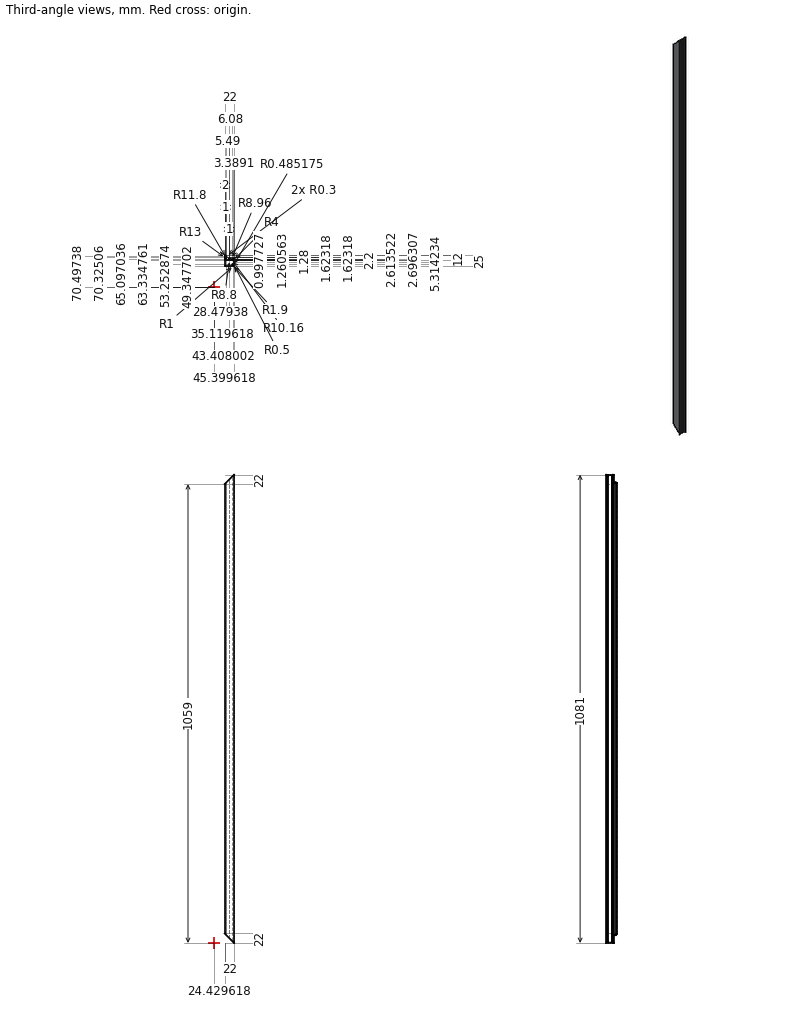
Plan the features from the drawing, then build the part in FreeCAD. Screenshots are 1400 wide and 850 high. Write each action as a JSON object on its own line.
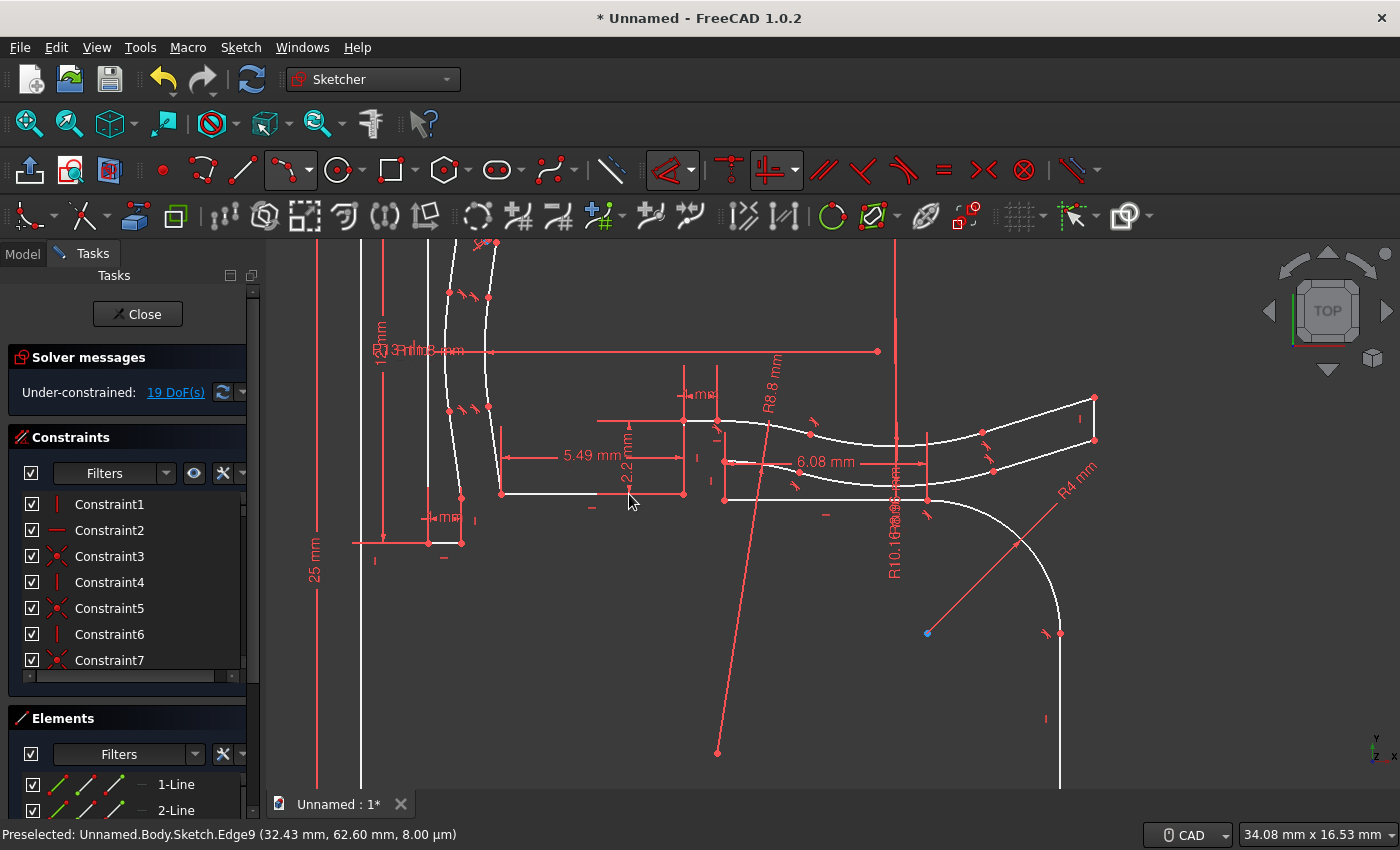
{"action": "left_click", "coordinate": [461, 530]}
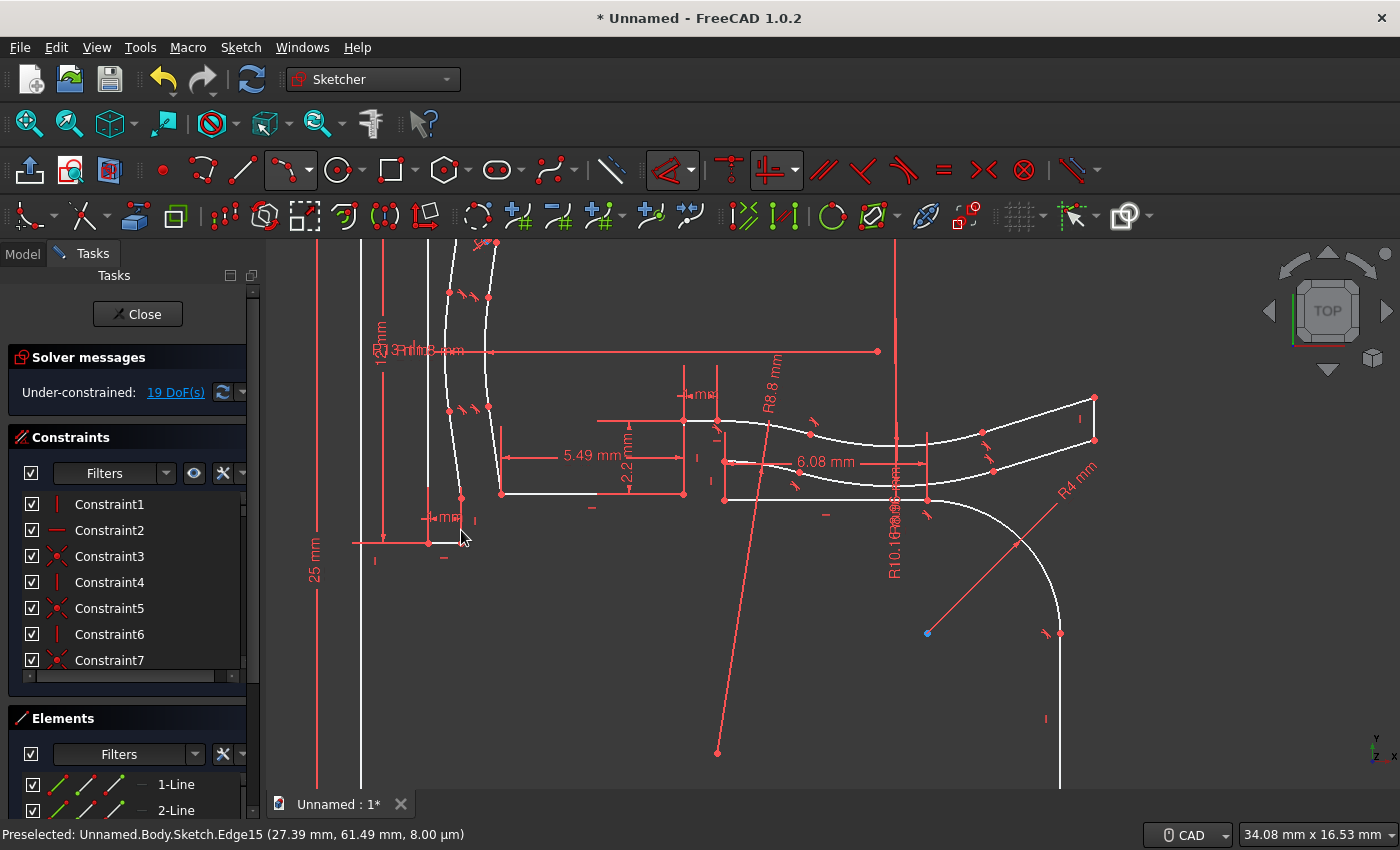
{"action": "left_click", "coordinate": [694, 170]}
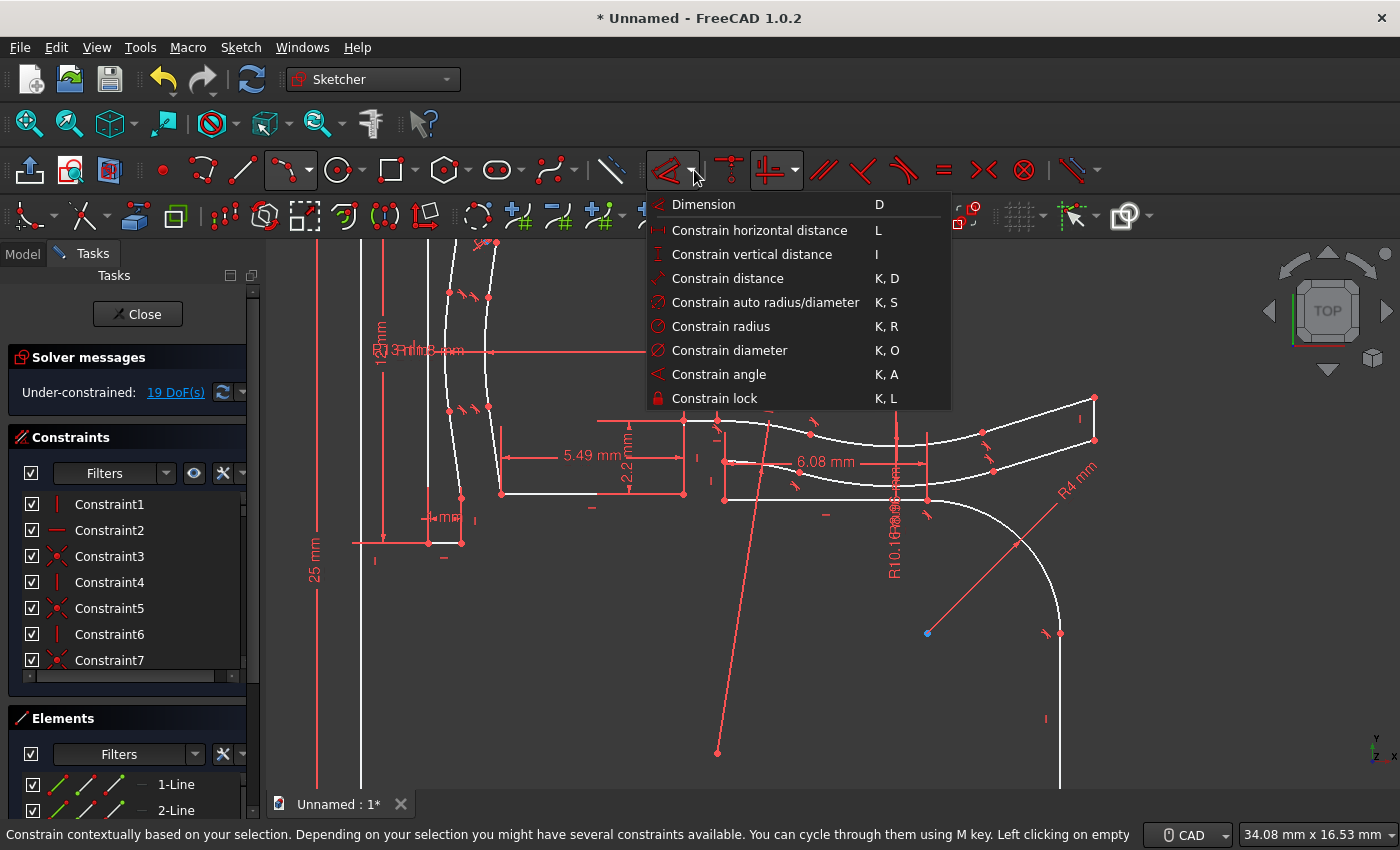
{"action": "left_click", "coordinate": [799, 254]}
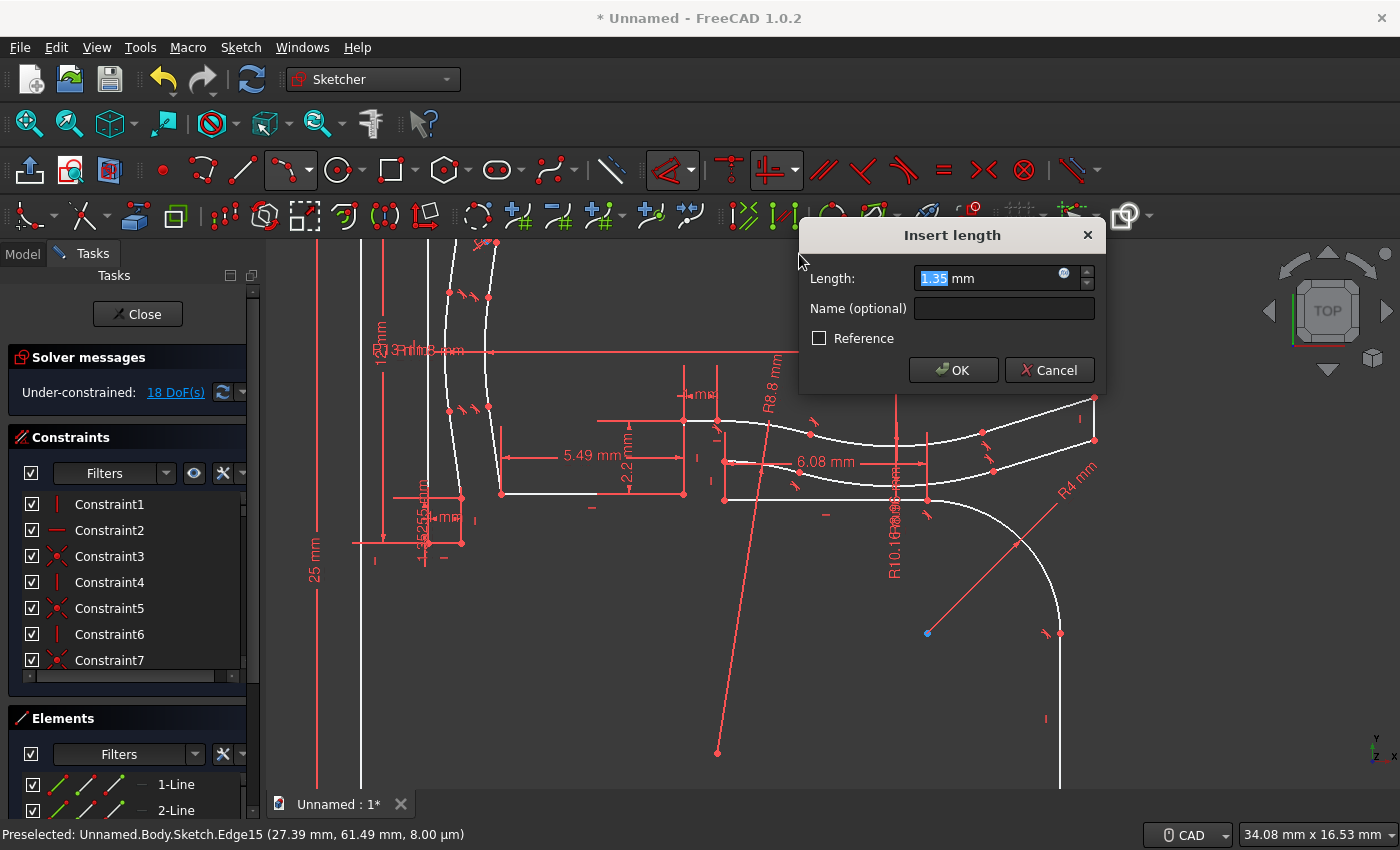
{"action": "type", "text": "1.28"}
{"action": "key", "text": "Return"}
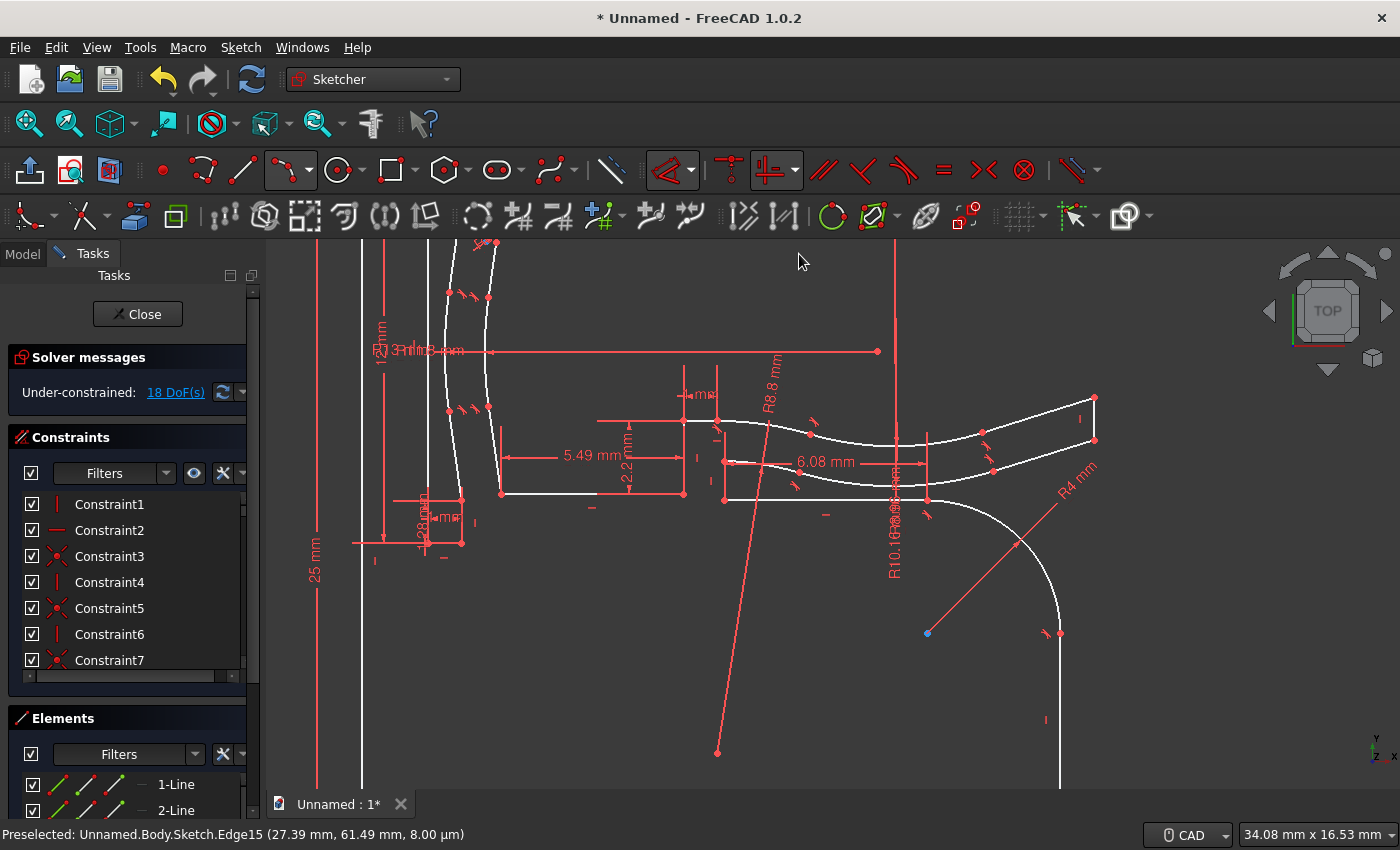
{"action": "left_click", "coordinate": [1061, 408]}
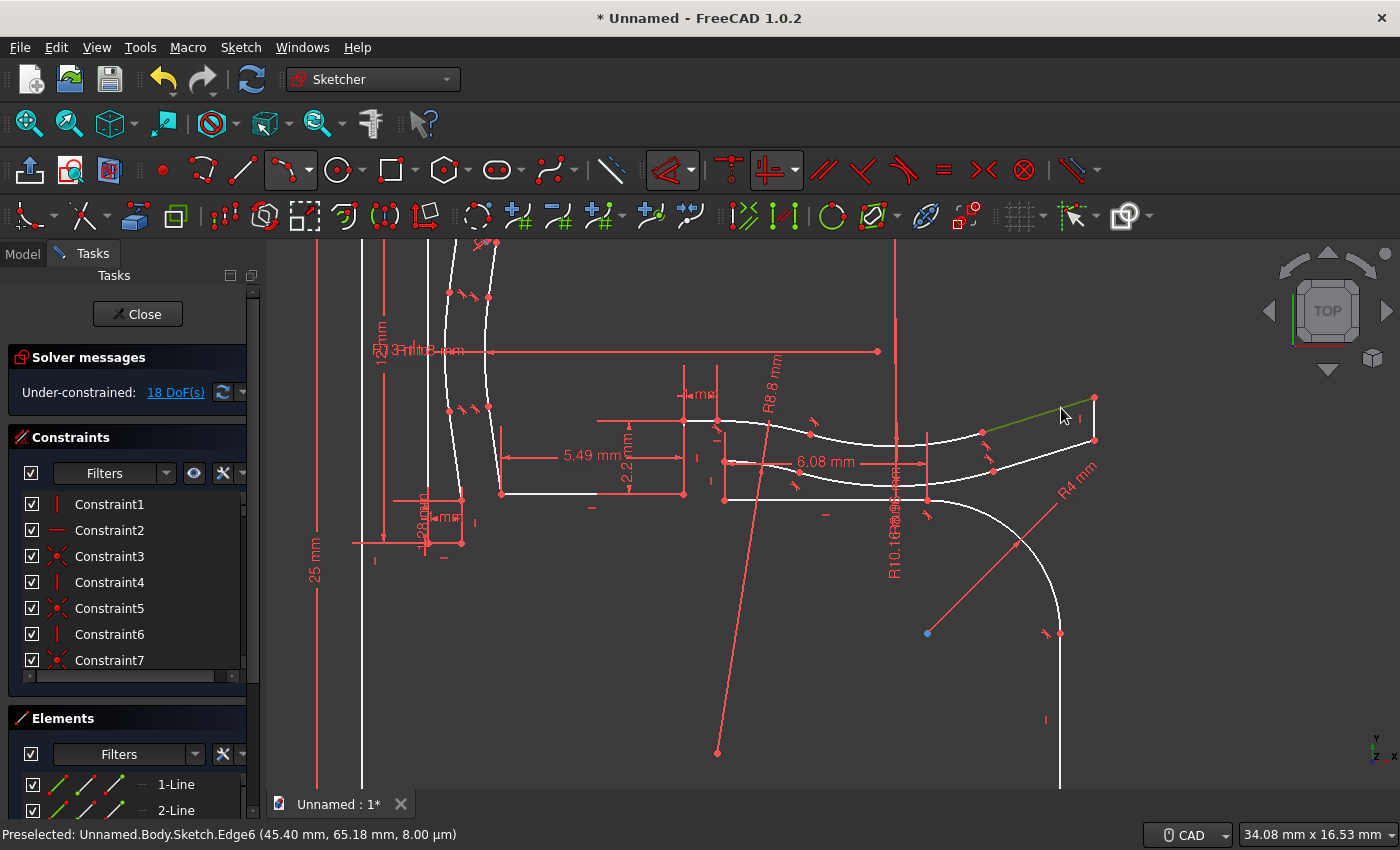
{"action": "left_click", "coordinate": [694, 170]}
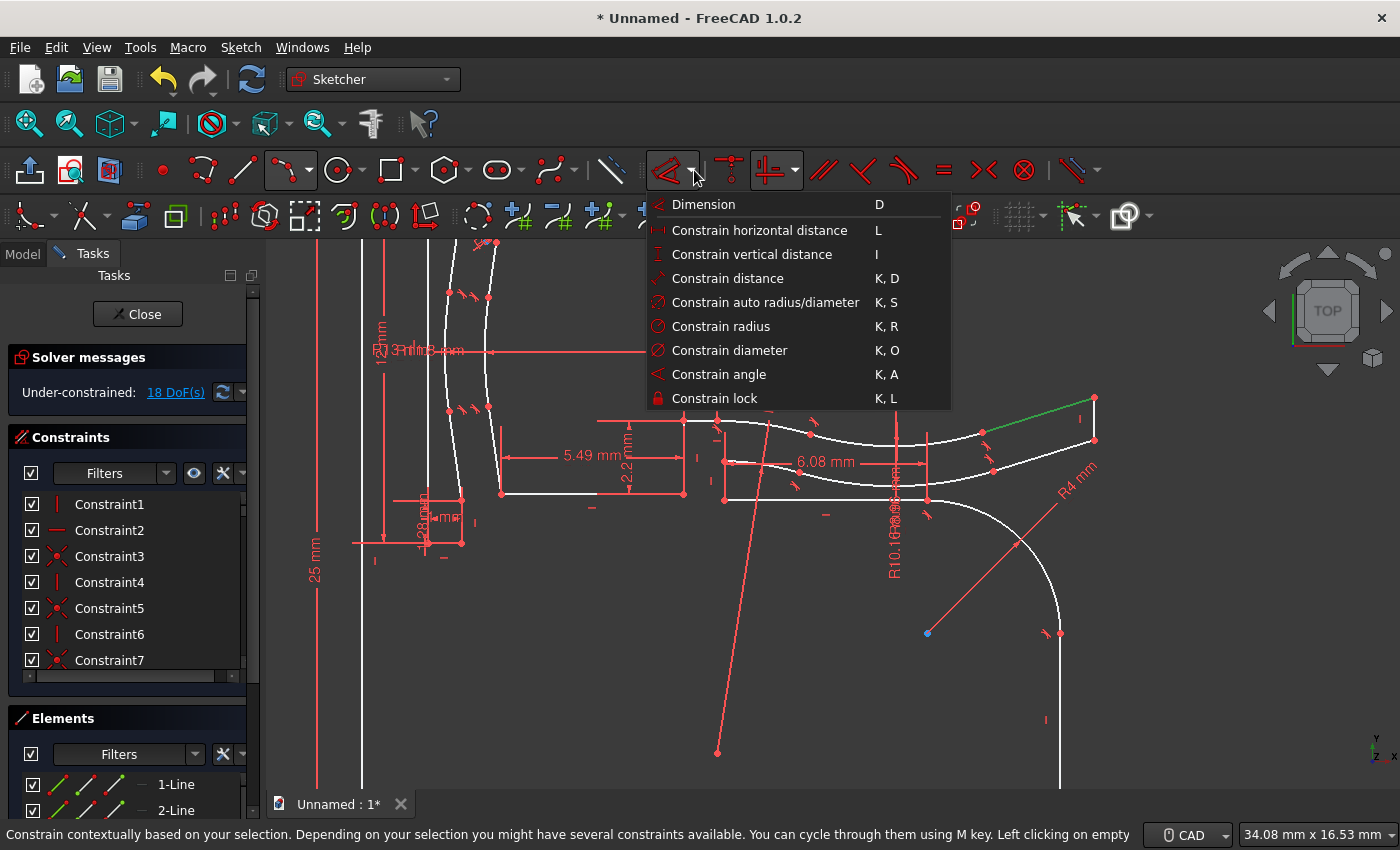
{"action": "left_click", "coordinate": [799, 230]}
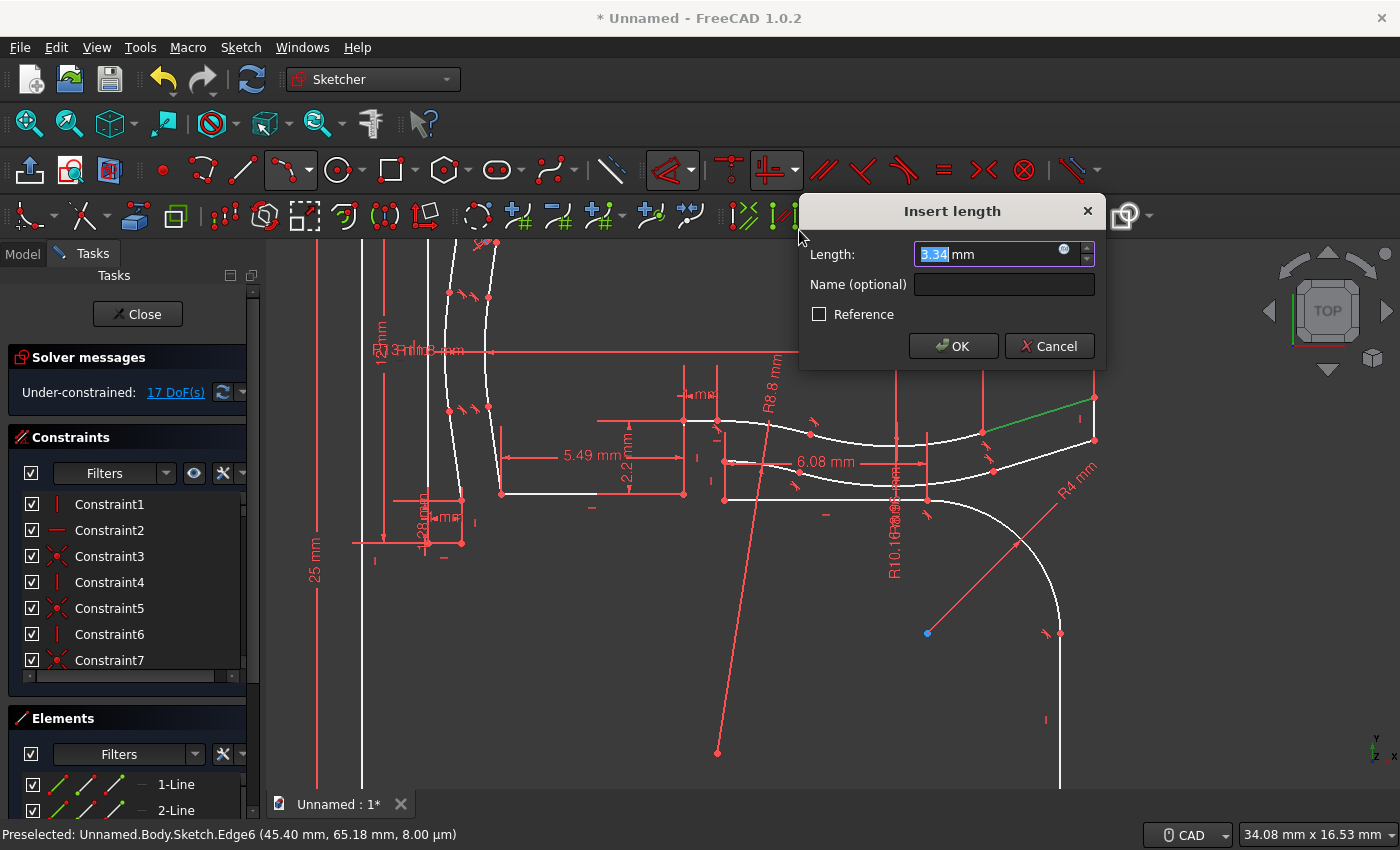
{"action": "type", "text": "3.3891"}
{"action": "key", "text": "Return"}